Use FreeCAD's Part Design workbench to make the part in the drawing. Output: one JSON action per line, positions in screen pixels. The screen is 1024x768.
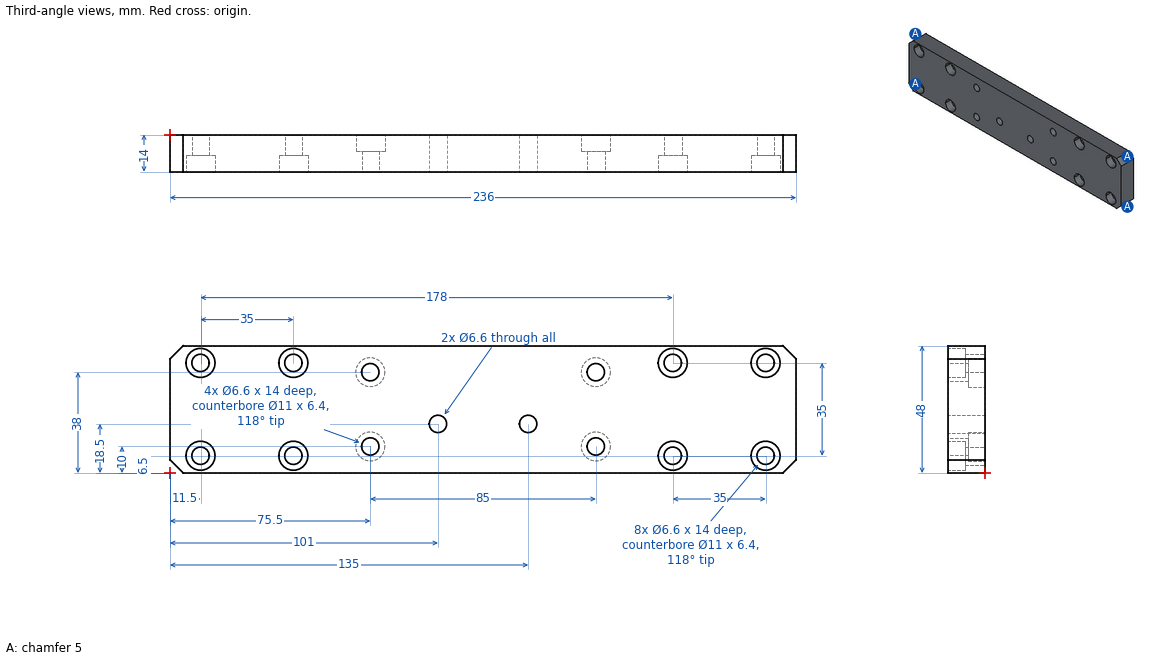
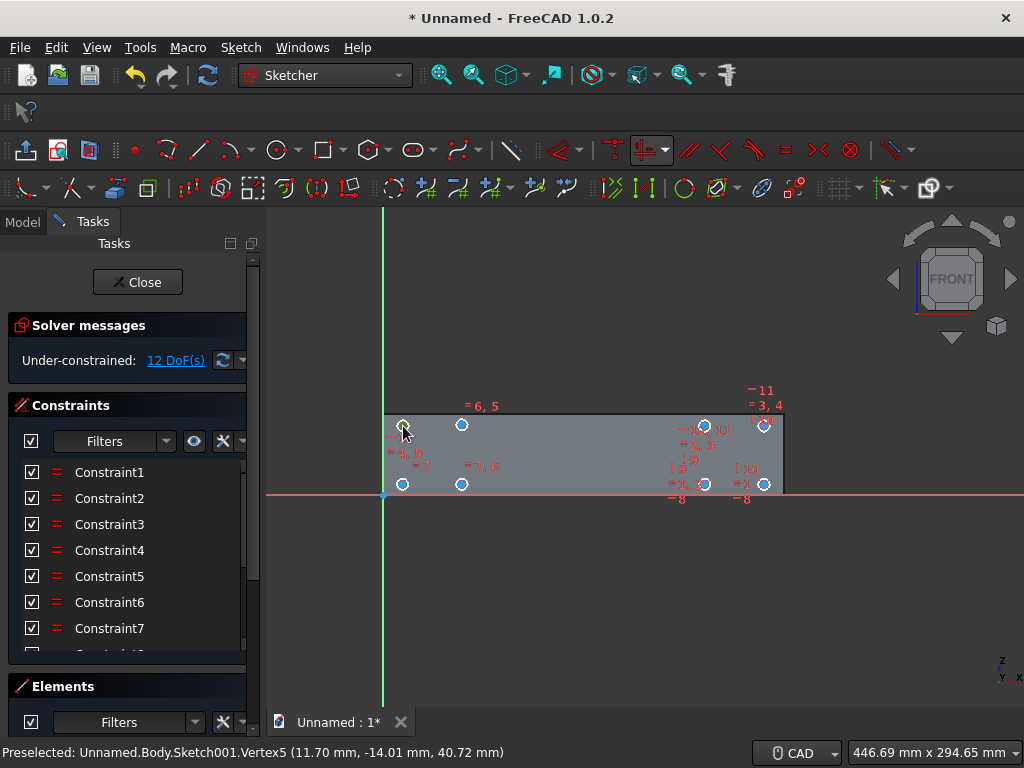
{"action": "left_click", "coordinate": [462, 425]}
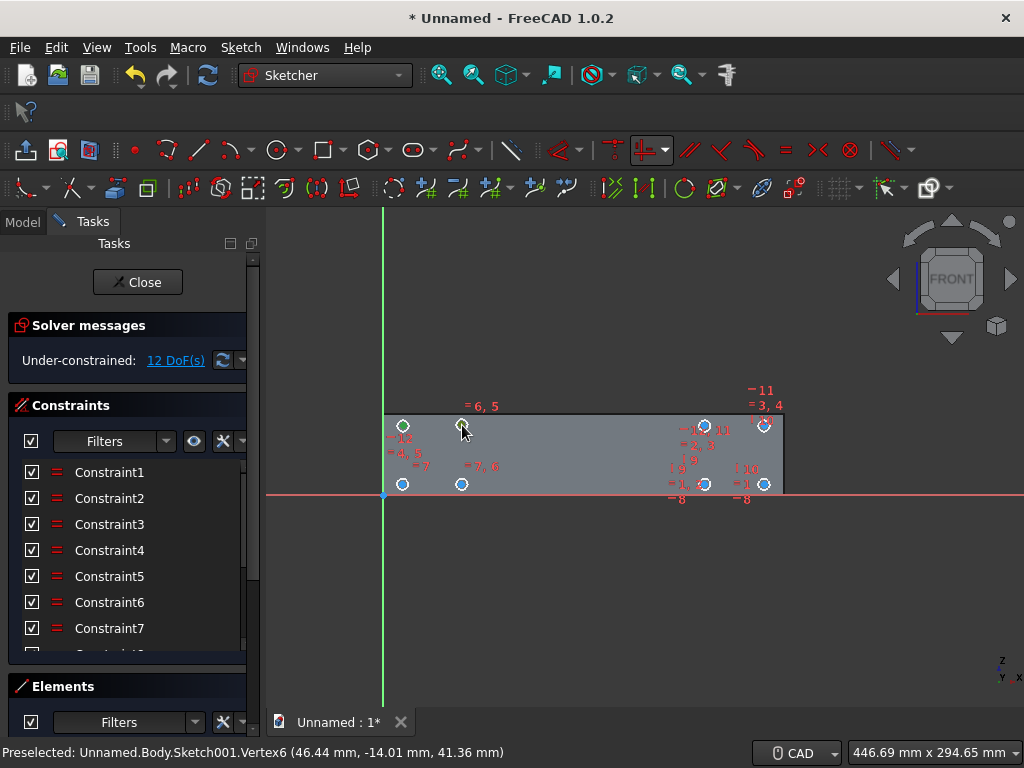
{"action": "left_click", "coordinate": [668, 150]}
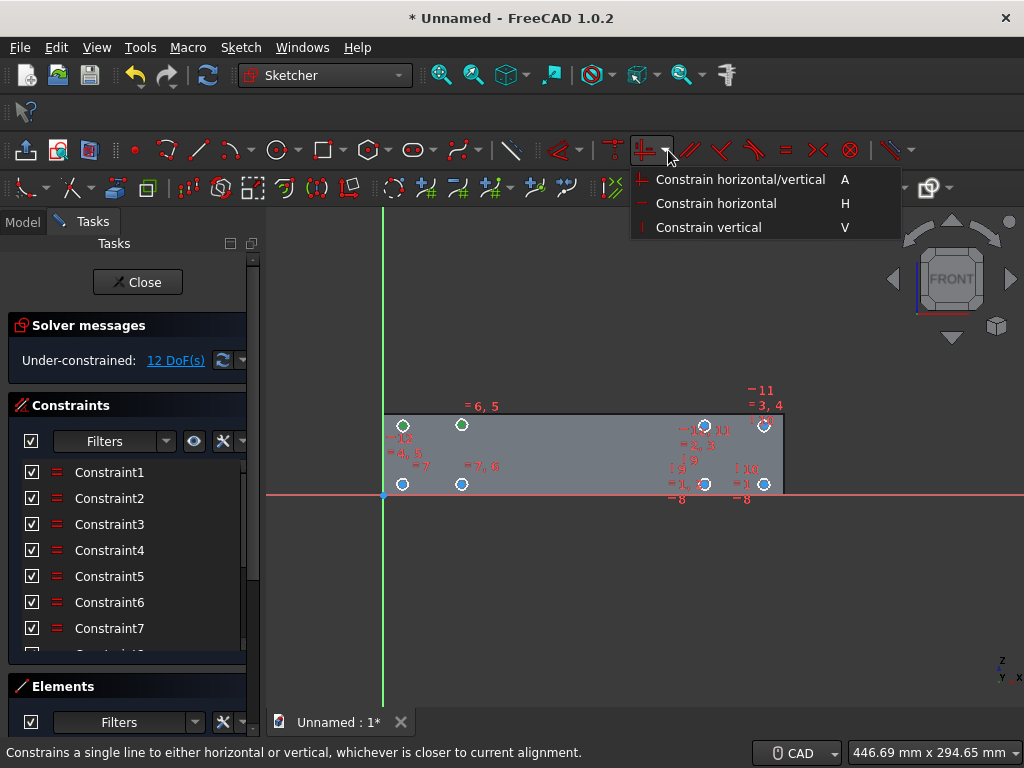
{"action": "left_click", "coordinate": [766, 203]}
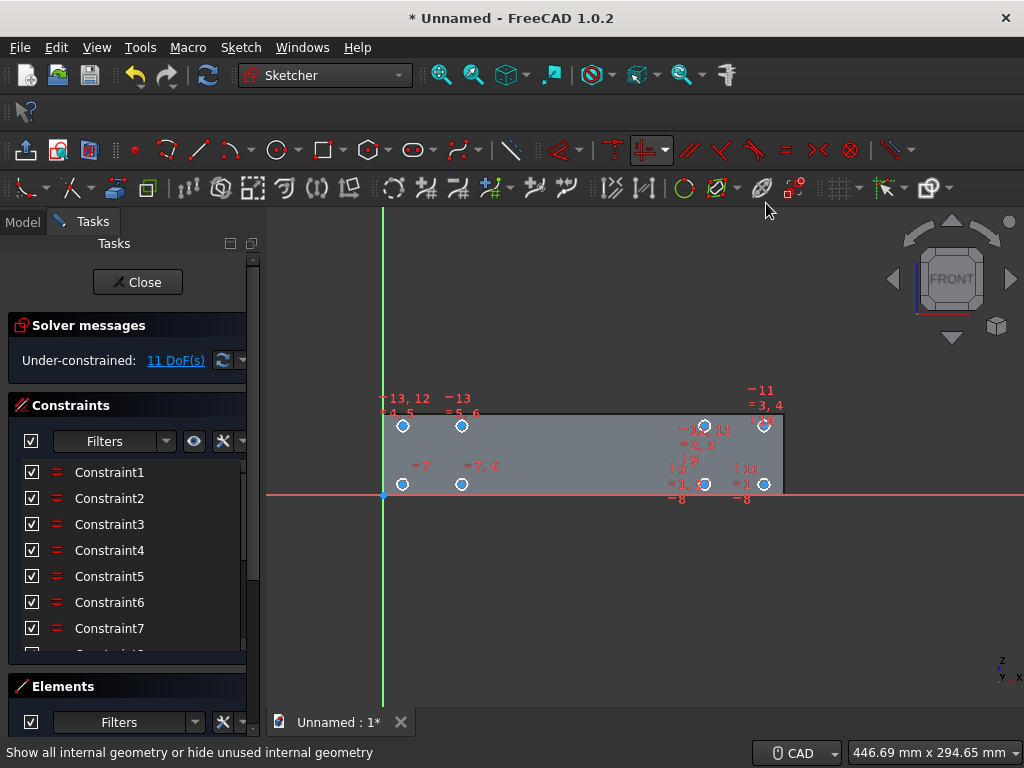
{"action": "left_click", "coordinate": [462, 426]}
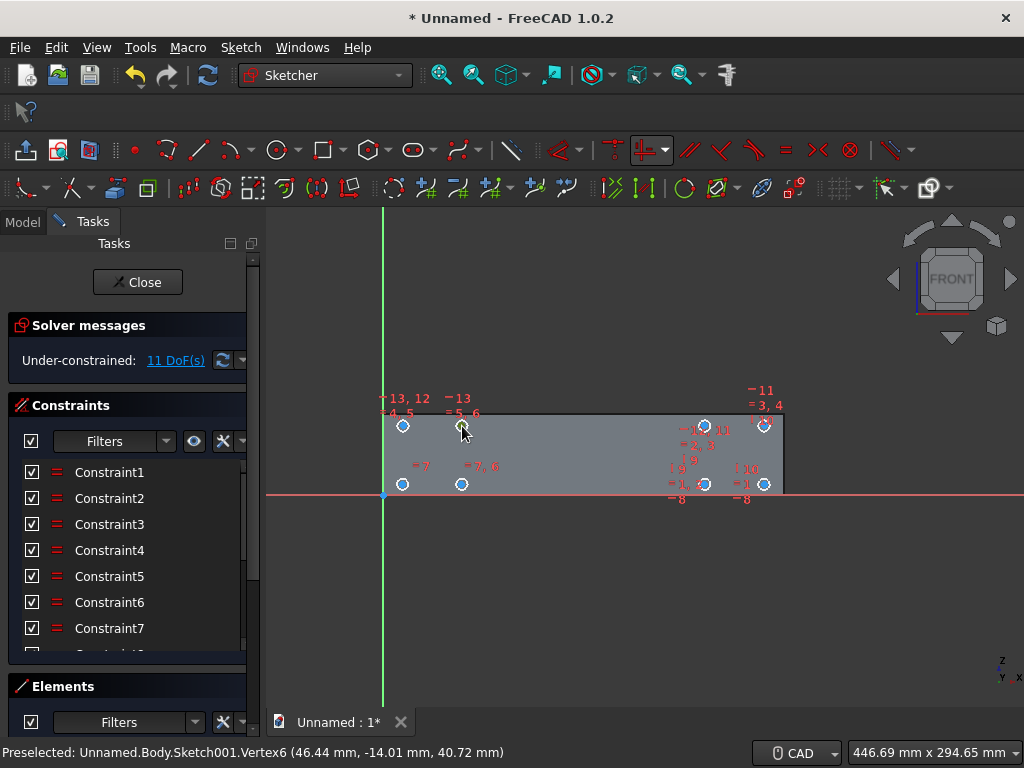
{"action": "left_click", "coordinate": [462, 484]}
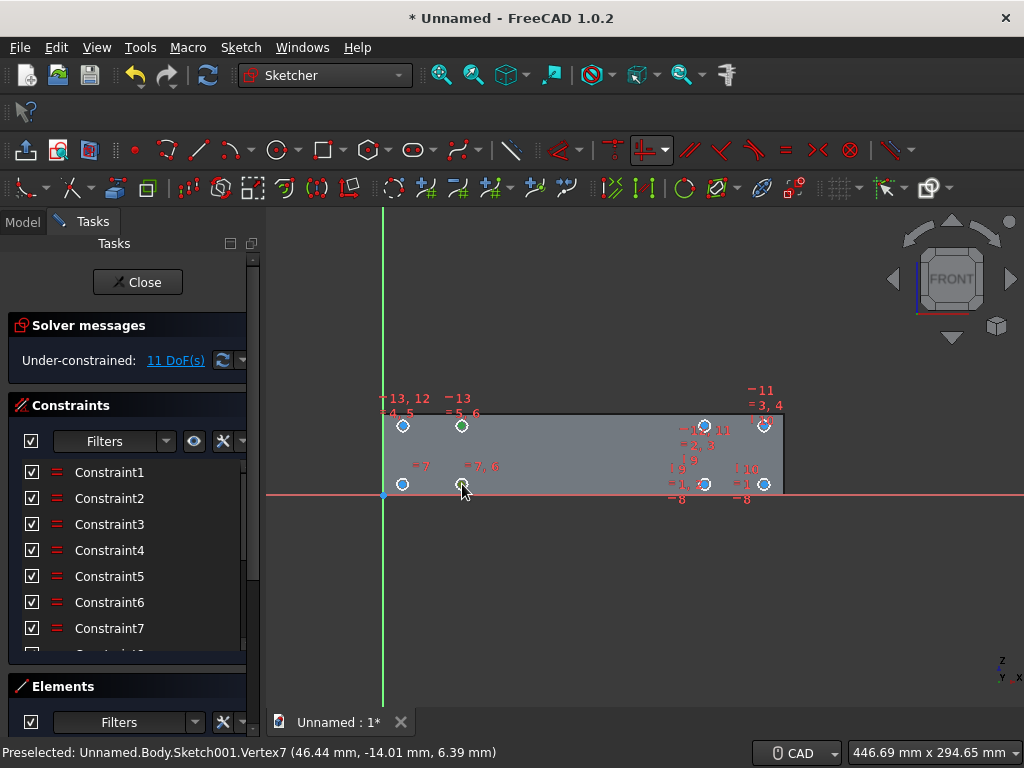
{"action": "key", "text": "v"}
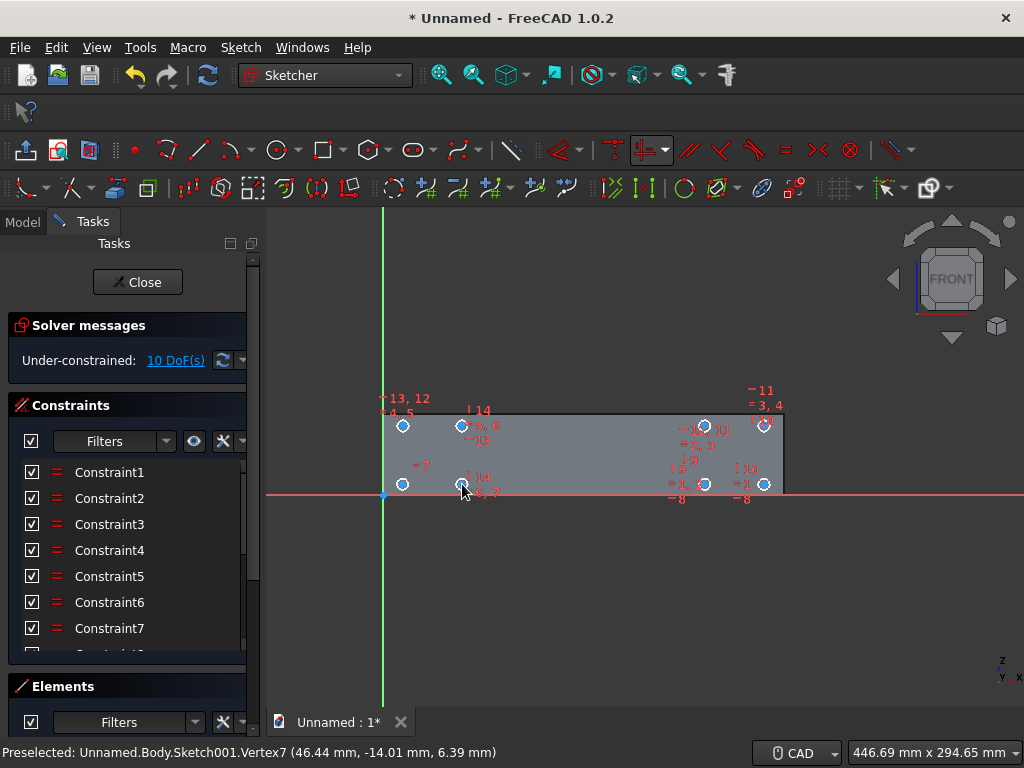
{"action": "left_click", "coordinate": [705, 484]}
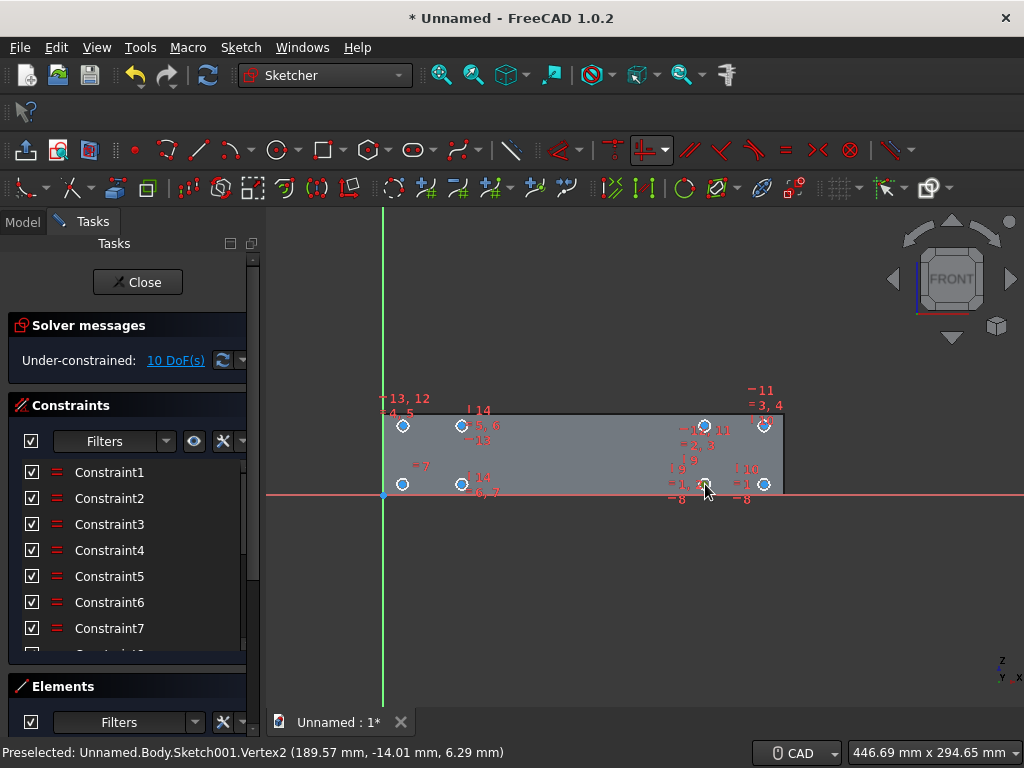
{"action": "left_click", "coordinate": [462, 484]}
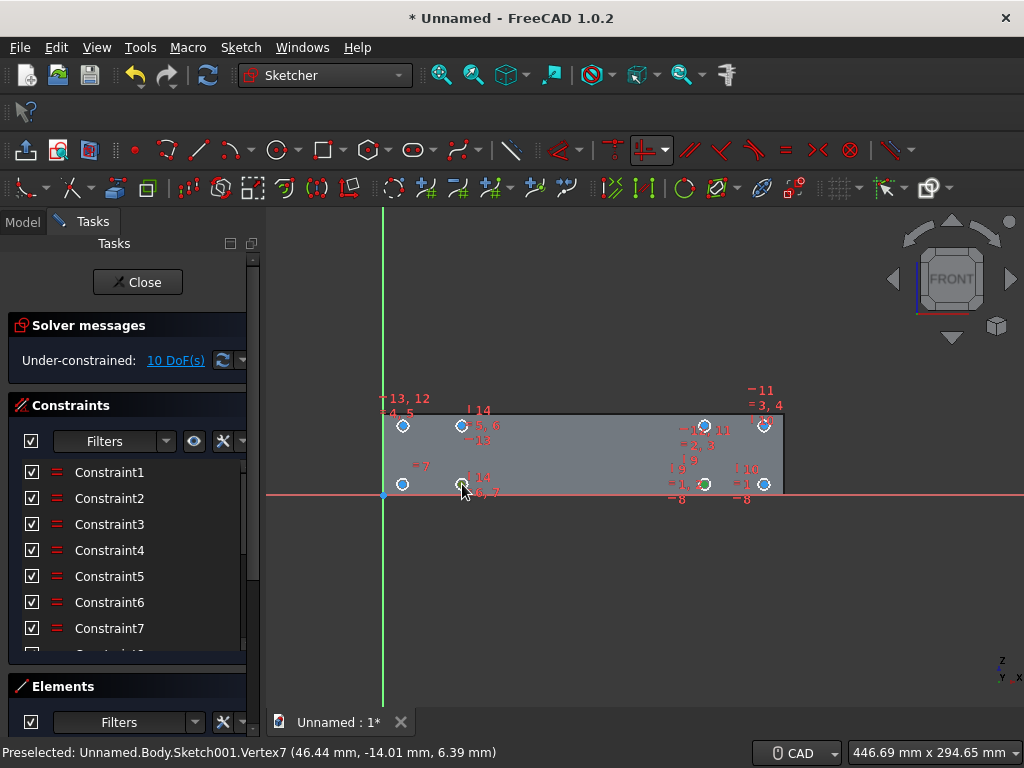
{"action": "left_click", "coordinate": [668, 150]}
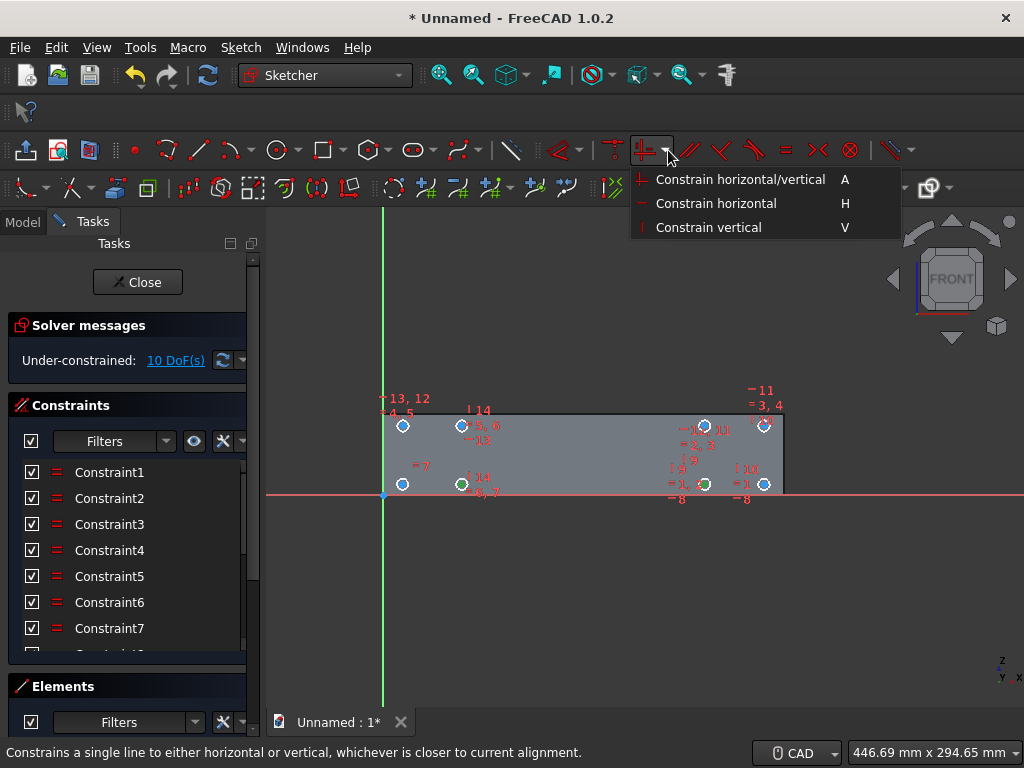
{"action": "left_click", "coordinate": [766, 203]}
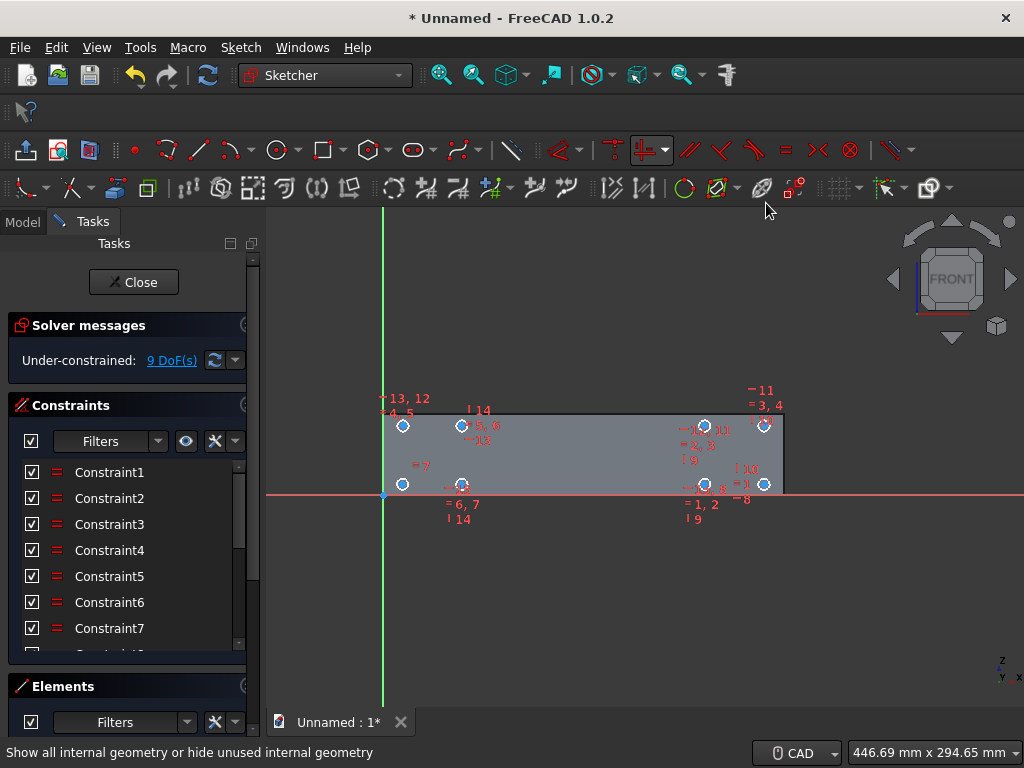
{"action": "left_click", "coordinate": [403, 426]}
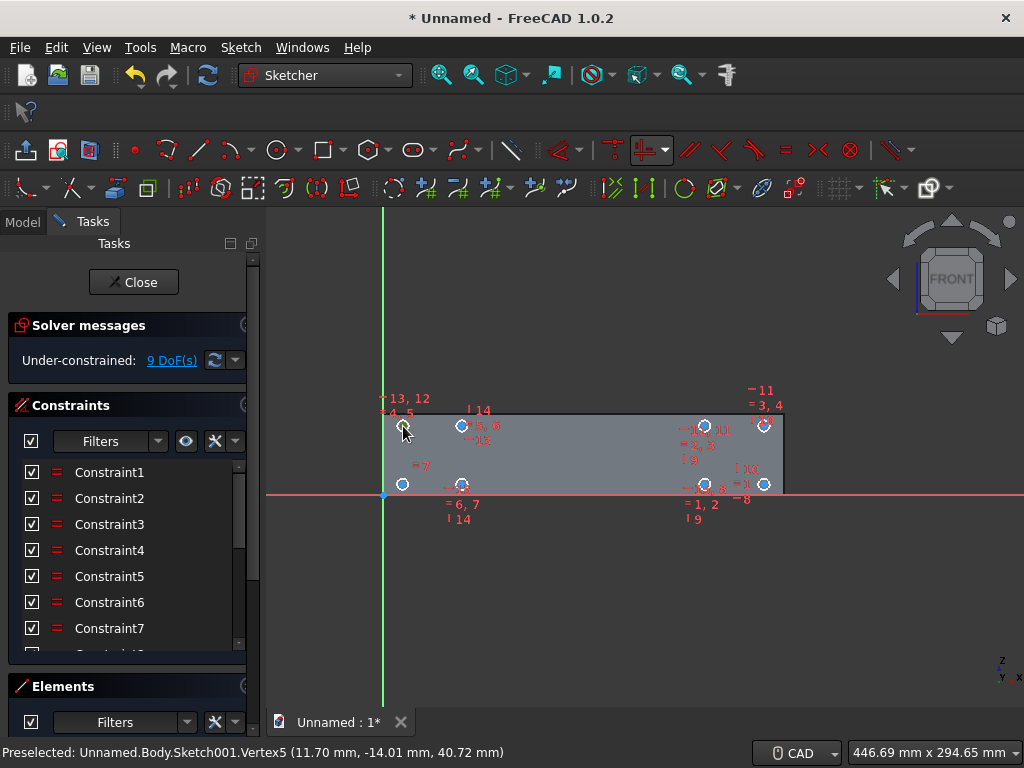
{"action": "left_click", "coordinate": [403, 484]}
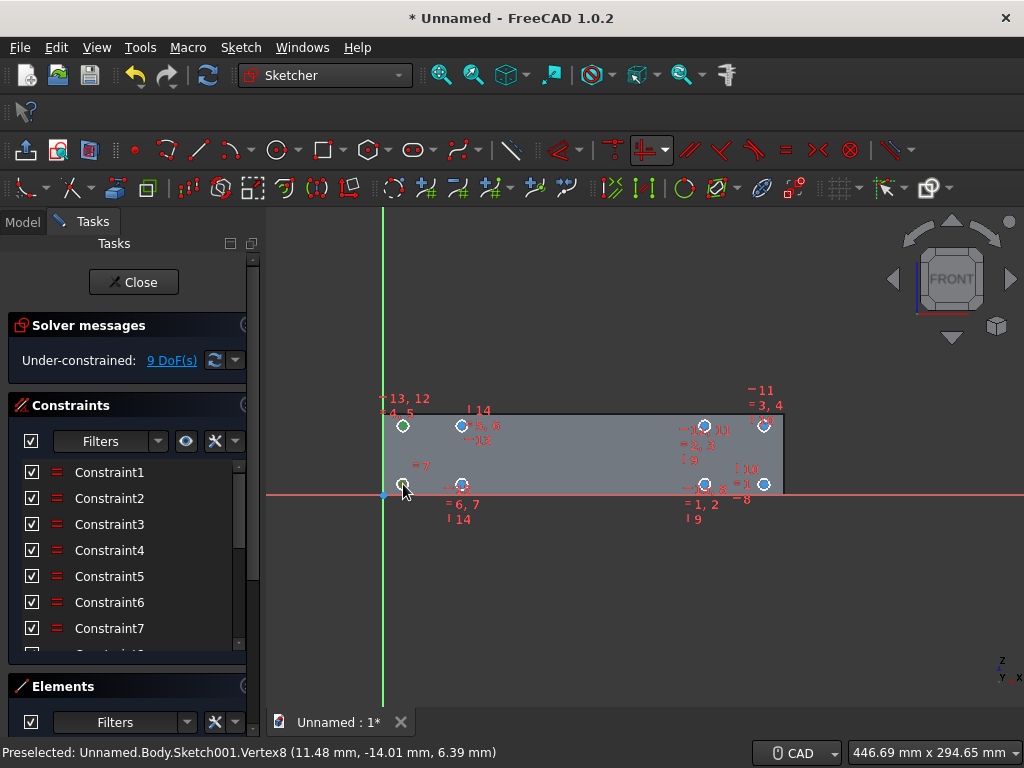
{"action": "key", "text": "v"}